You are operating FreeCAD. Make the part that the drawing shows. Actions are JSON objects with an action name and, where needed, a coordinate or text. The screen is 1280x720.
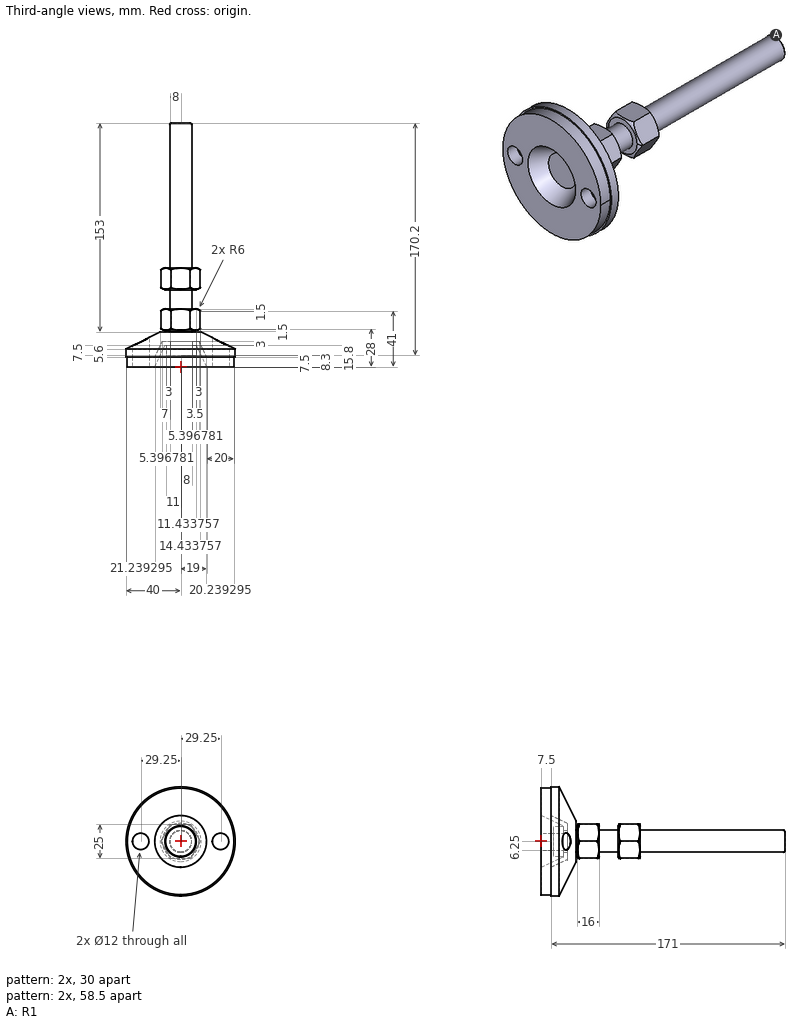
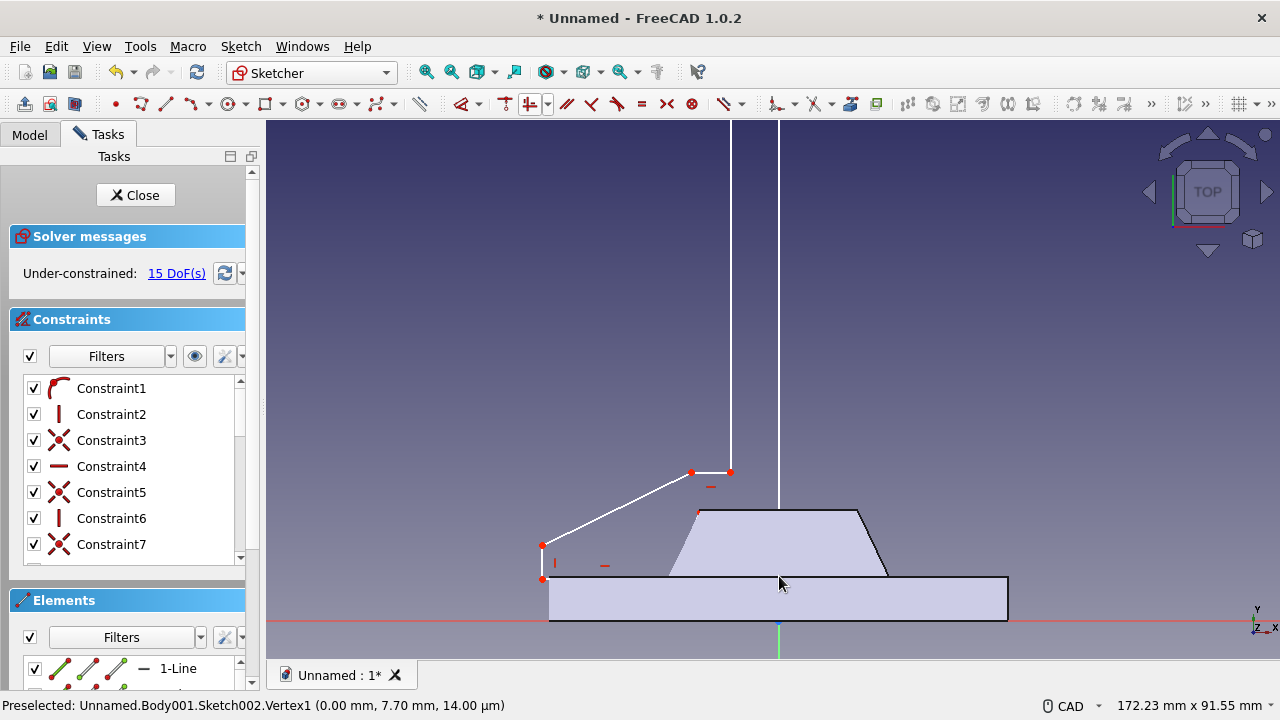
{"action": "left_click", "coordinate": [733, 574]}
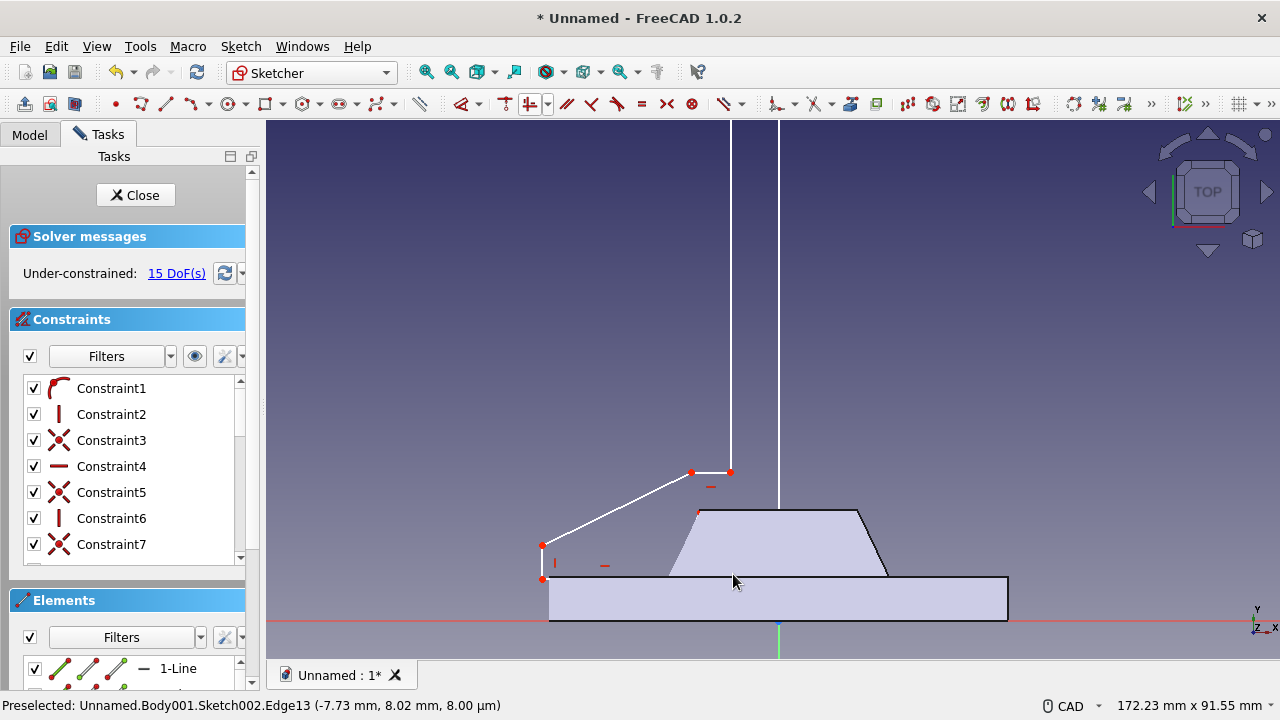
{"action": "key", "text": "h"}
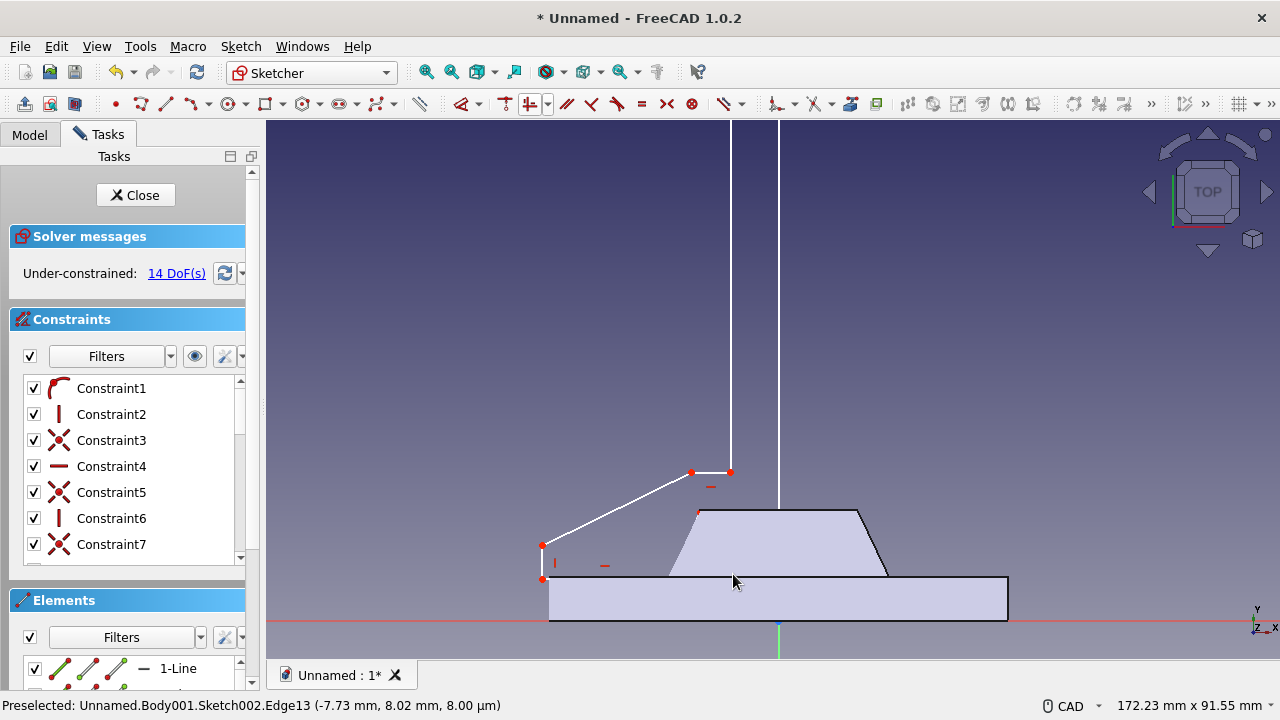
{"action": "left_click", "coordinate": [460, 104]}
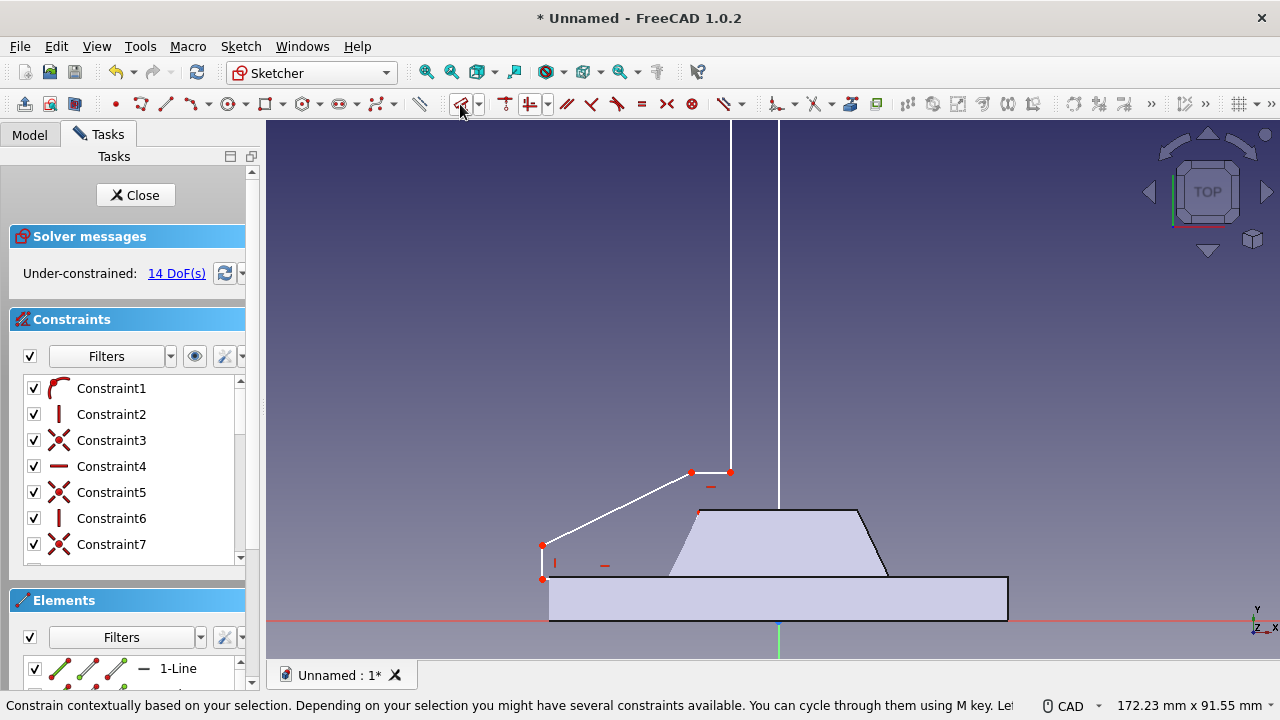
{"action": "scroll", "coordinate": [723, 516], "scroll_direction": "down", "scroll_amount": 6}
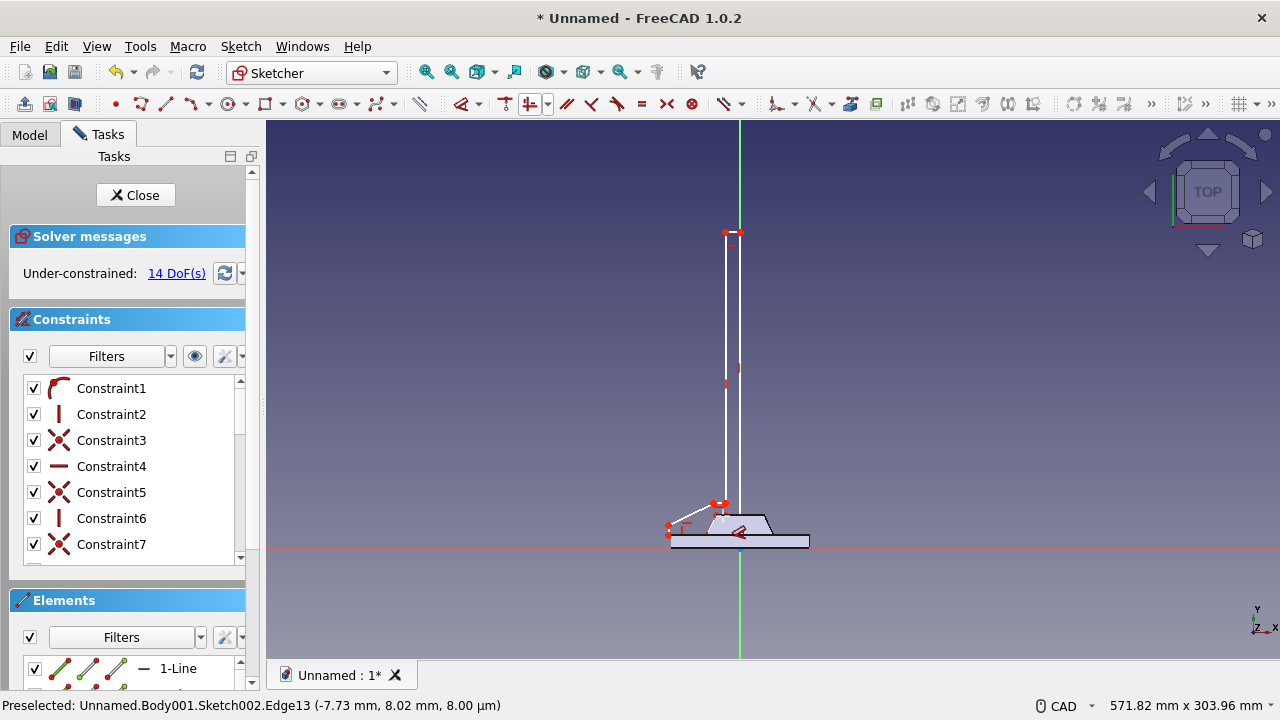
{"action": "scroll", "coordinate": [736, 232], "scroll_direction": "up", "scroll_amount": 6}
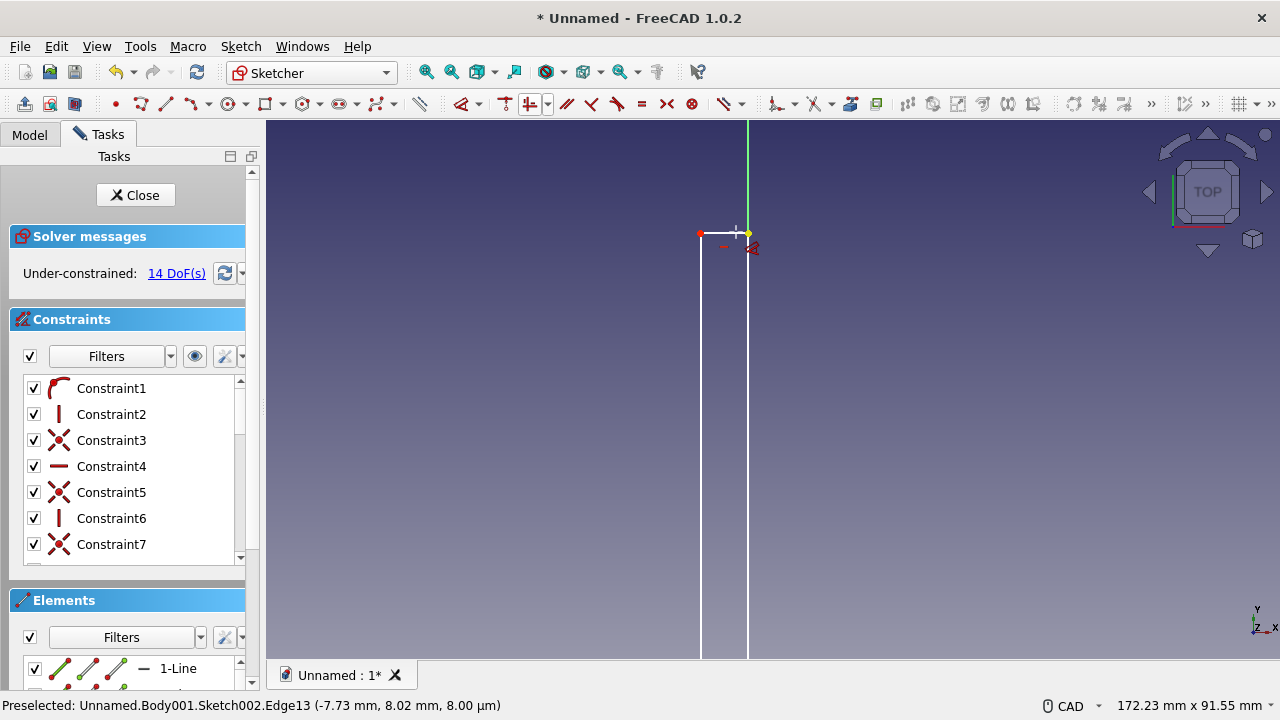
{"action": "left_click", "coordinate": [734, 233]}
{"action": "left_click", "coordinate": [724, 199]}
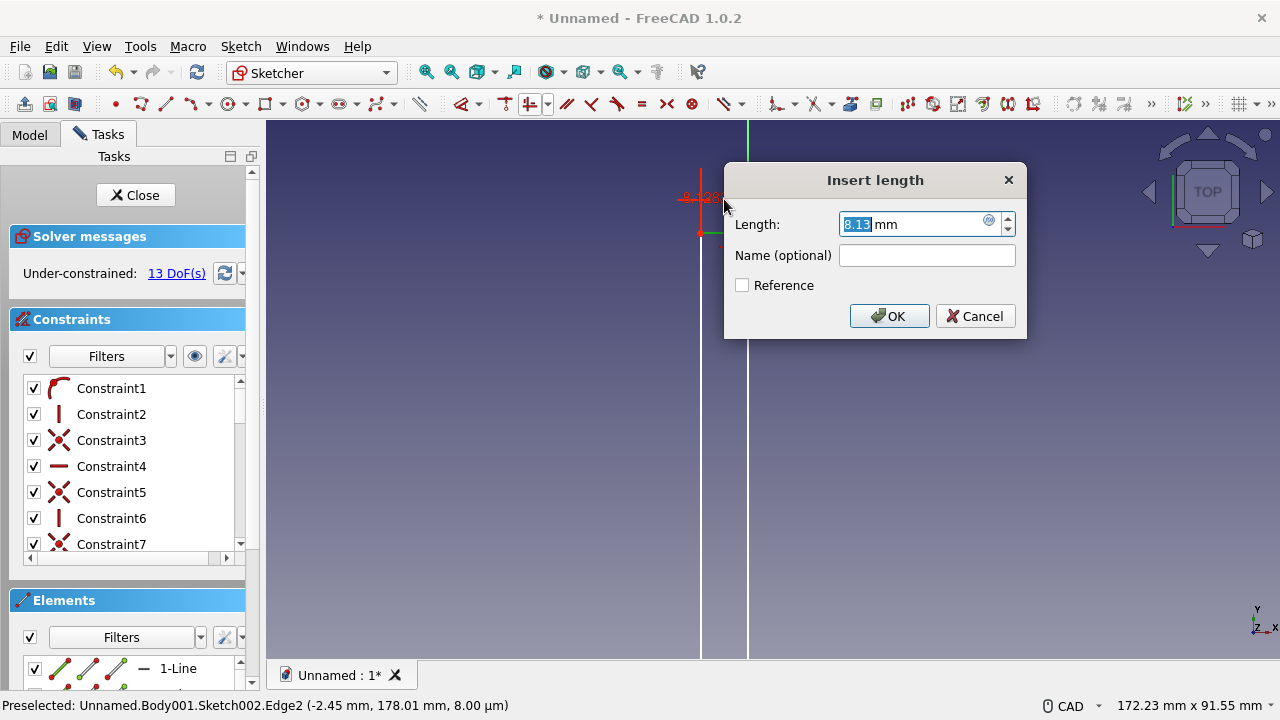
{"action": "type", "text": "8"}
{"action": "key", "text": "Return"}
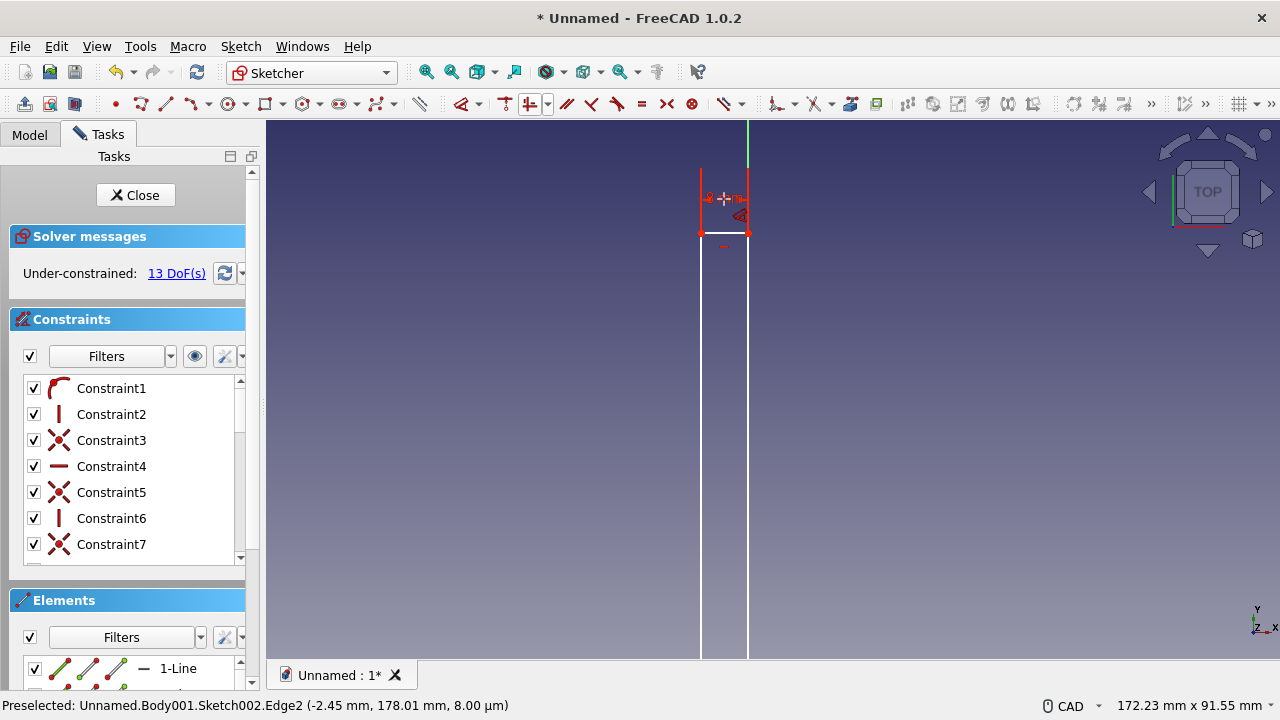
{"action": "scroll", "coordinate": [736, 232], "scroll_direction": "down", "scroll_amount": 6}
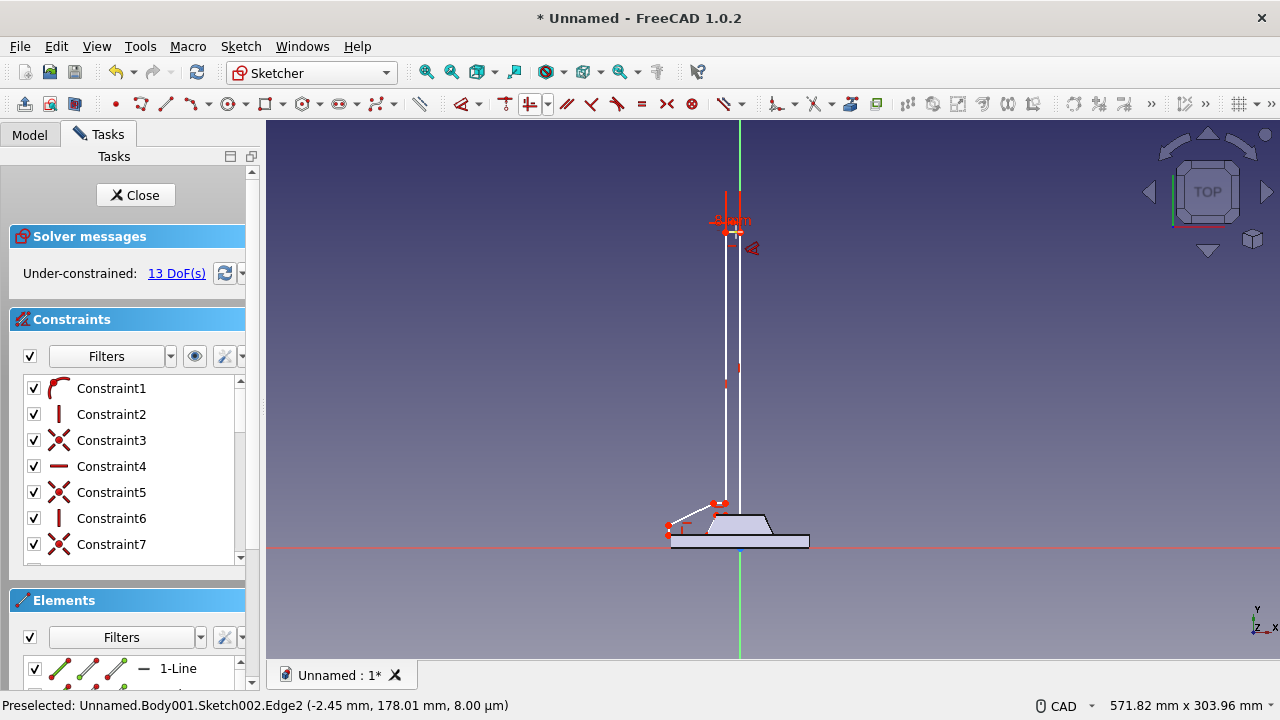
{"action": "scroll", "coordinate": [722, 503], "scroll_direction": "up", "scroll_amount": 7}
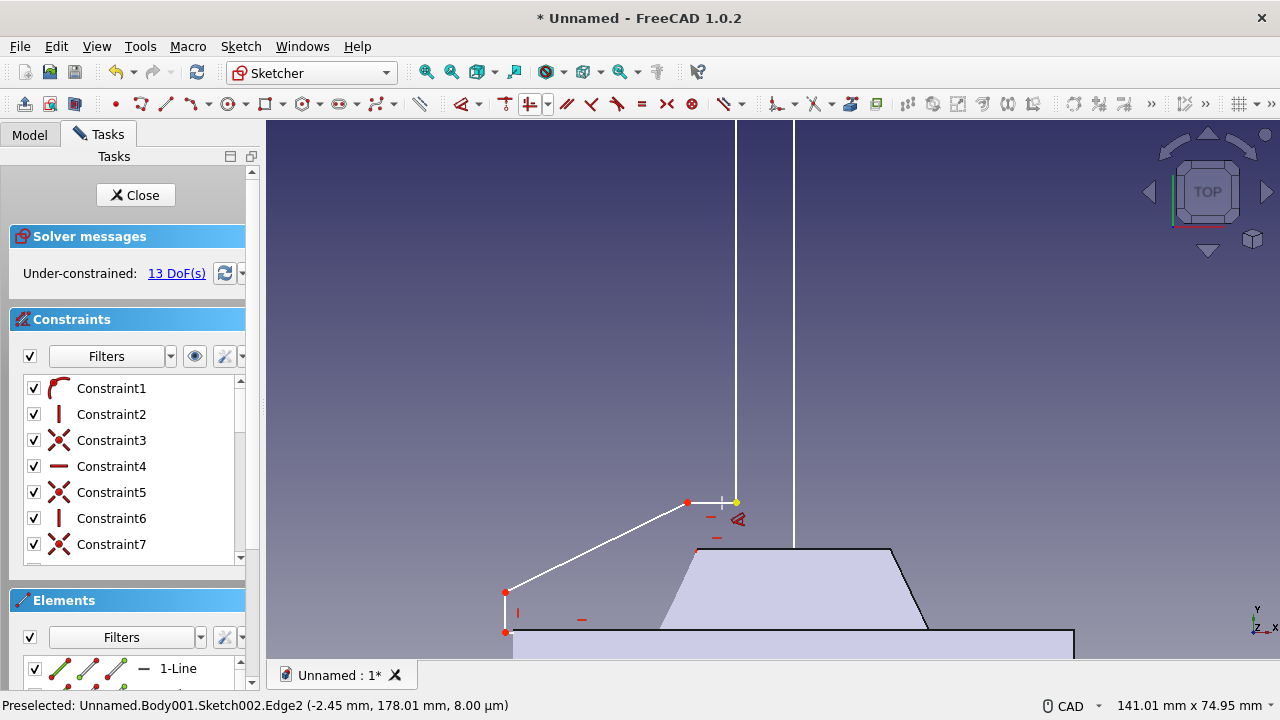
{"action": "left_click", "coordinate": [722, 503]}
{"action": "left_click", "coordinate": [712, 537]}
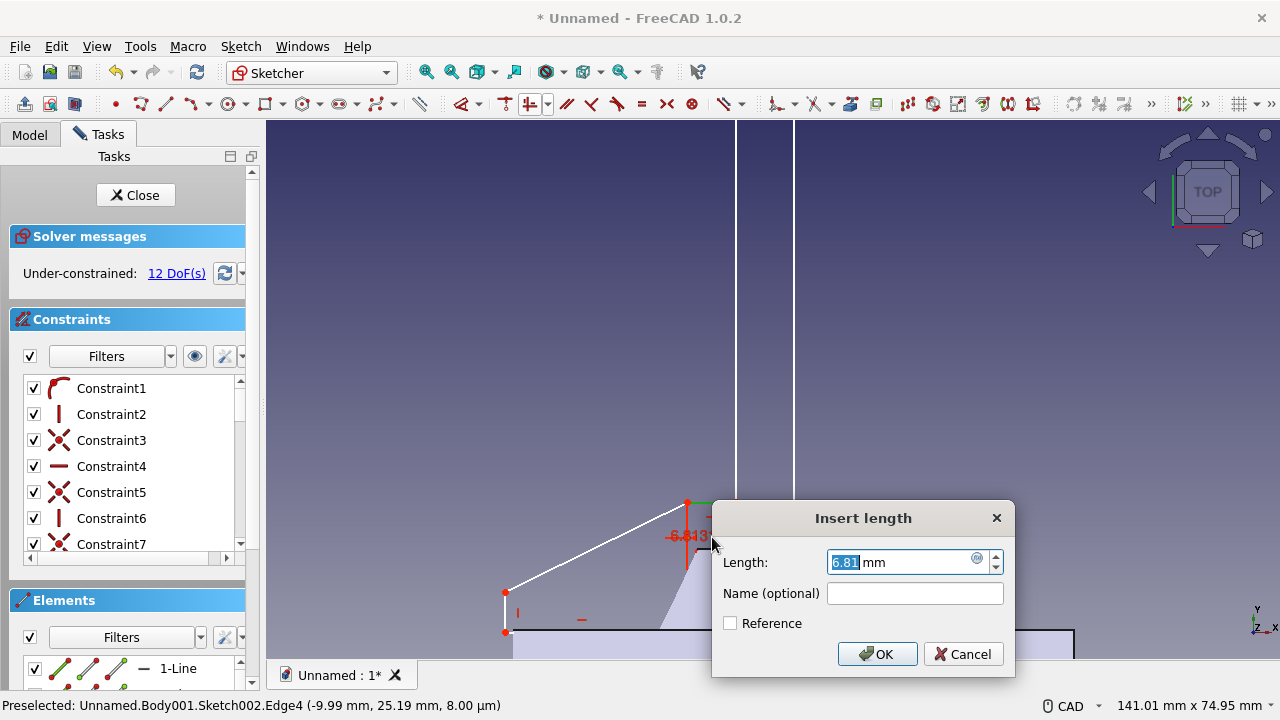
{"action": "type", "text": "7"}
{"action": "key", "text": "Return"}